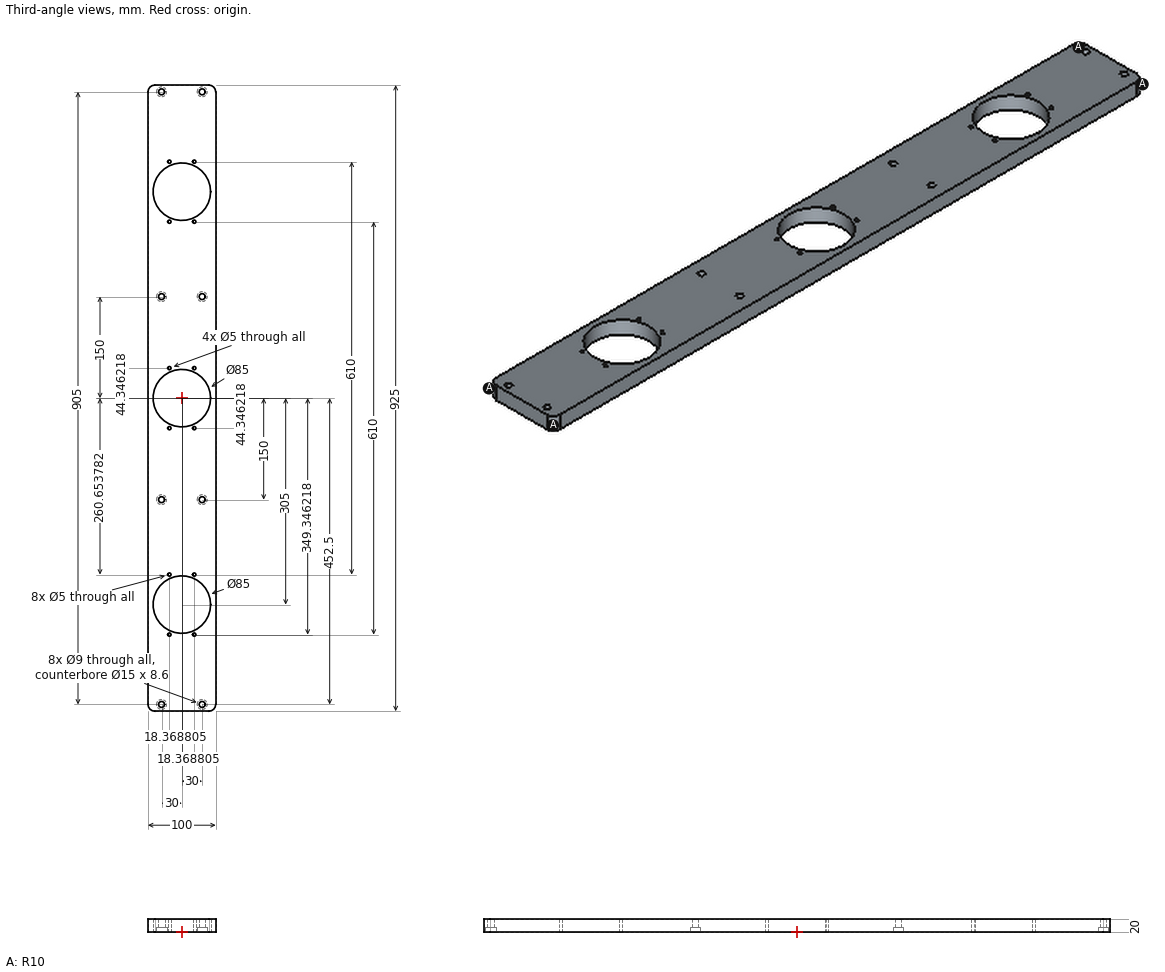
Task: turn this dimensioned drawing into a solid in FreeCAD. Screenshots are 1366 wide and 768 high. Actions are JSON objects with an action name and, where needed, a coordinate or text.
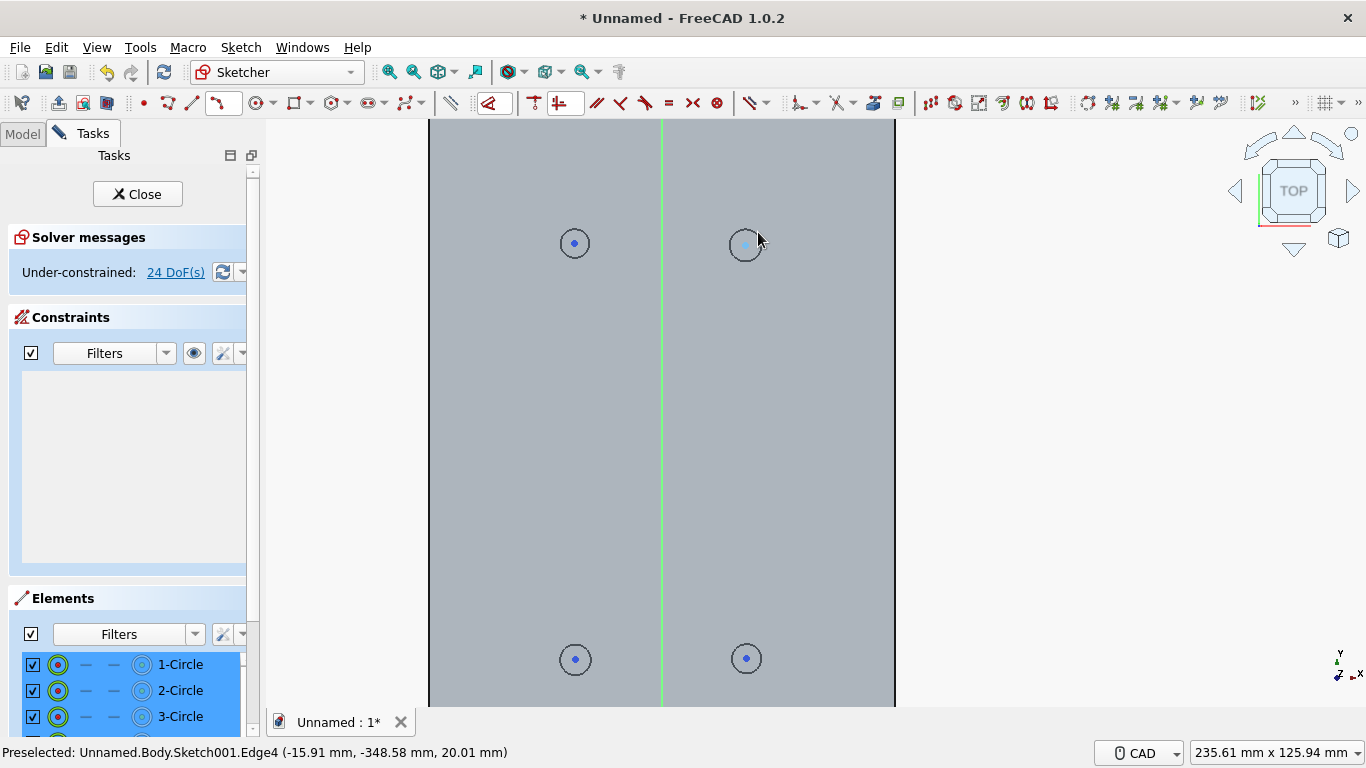
{"action": "left_click", "coordinate": [757, 234]}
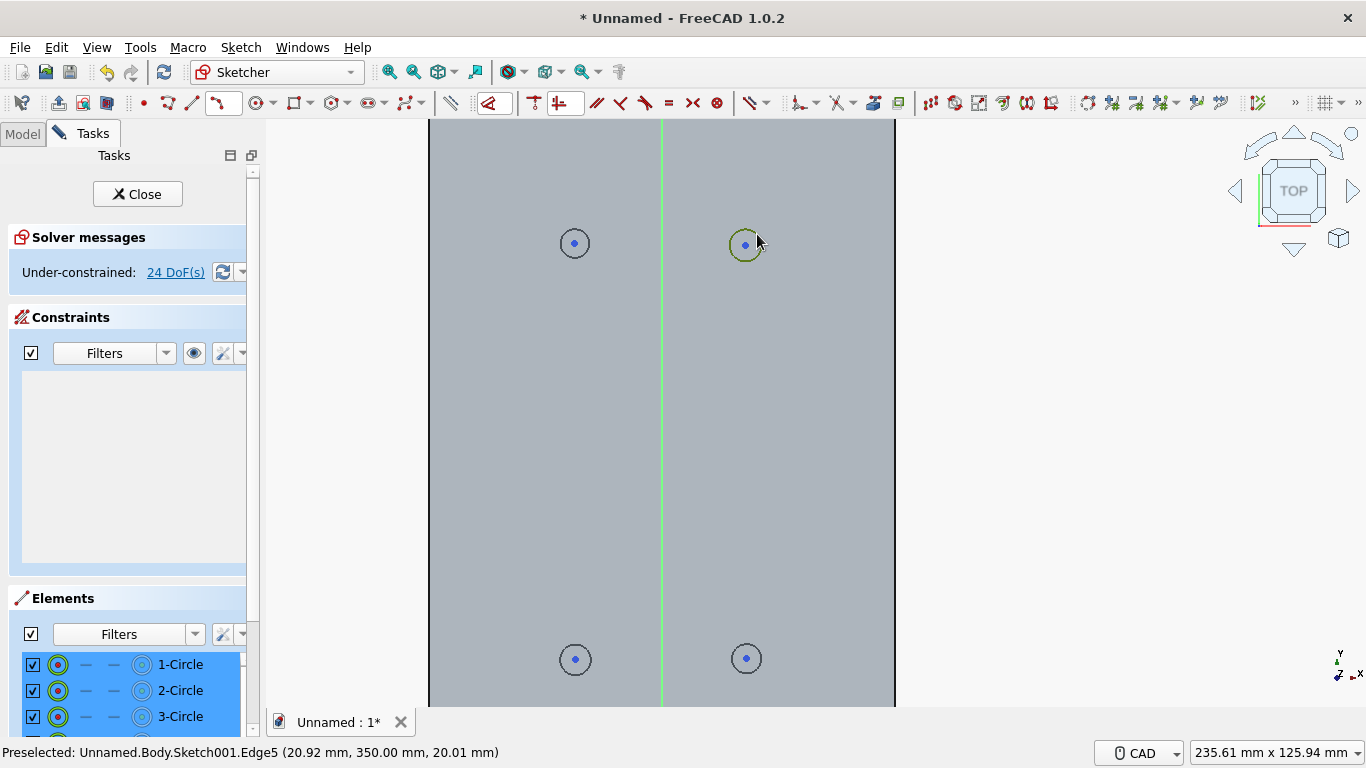
{"action": "left_click", "coordinate": [585, 233]}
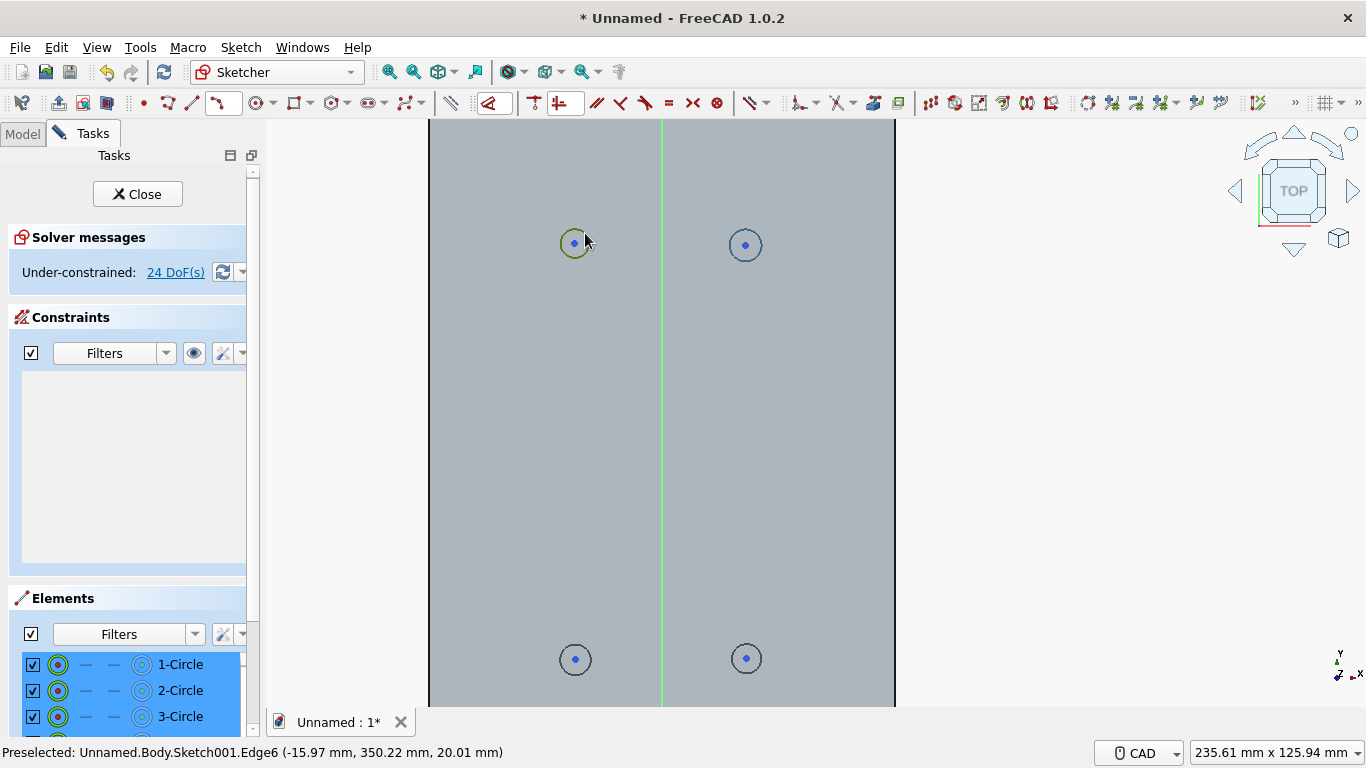
{"action": "left_click", "coordinate": [757, 648]}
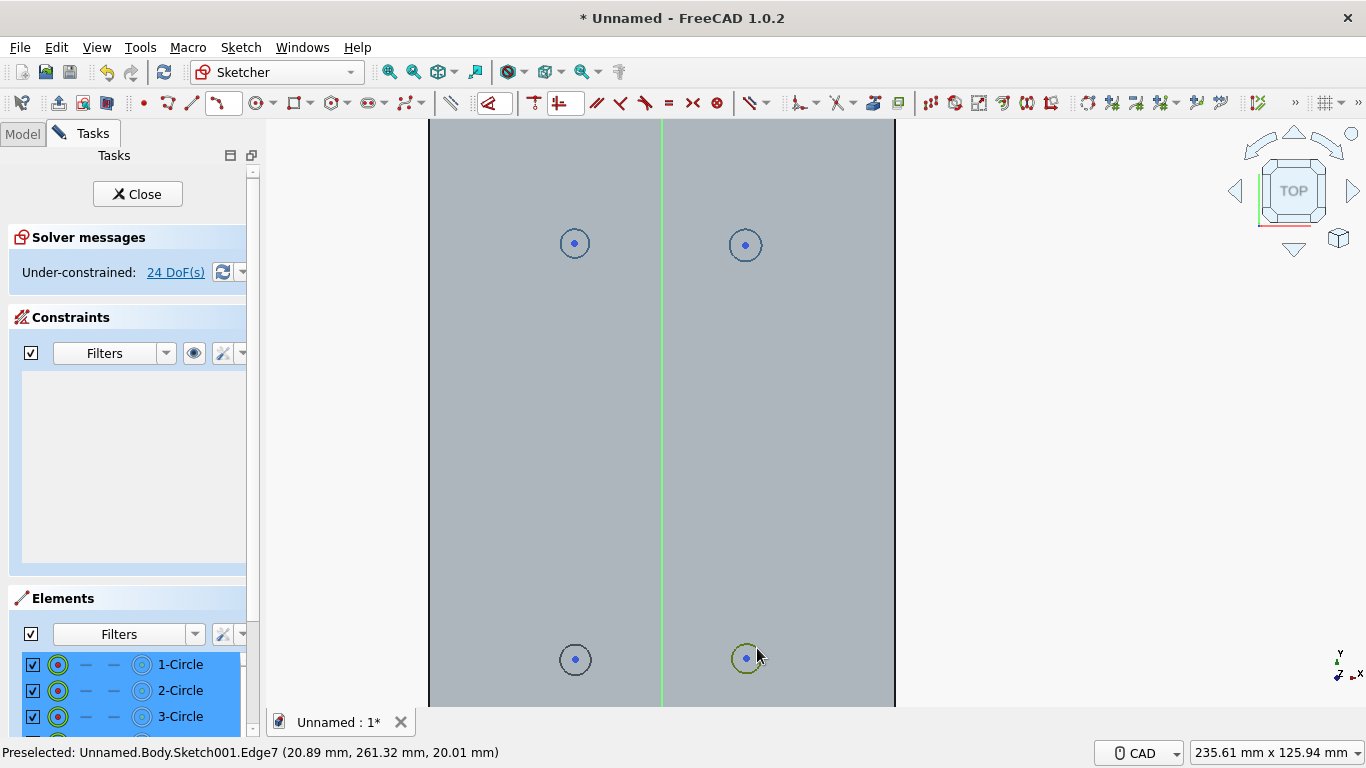
{"action": "left_click", "coordinate": [586, 649]}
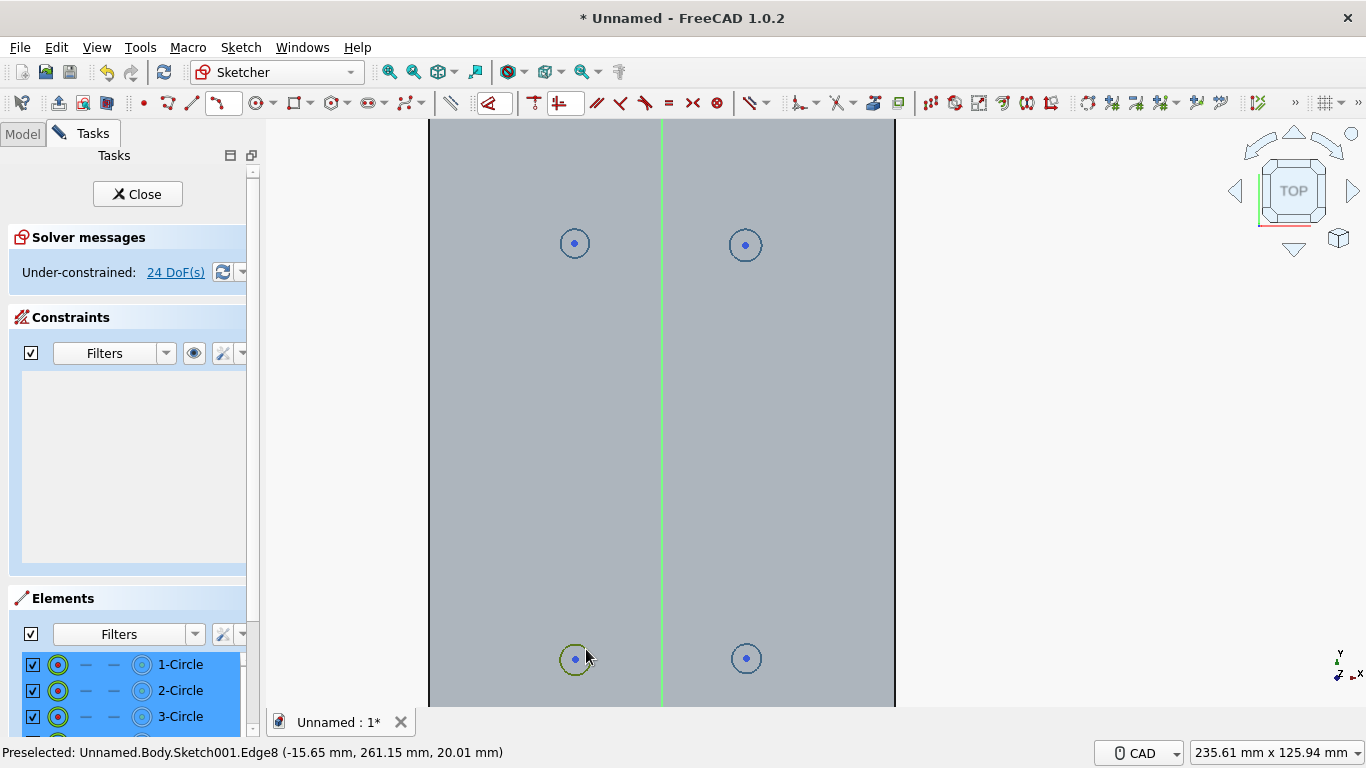
{"action": "key", "text": "e"}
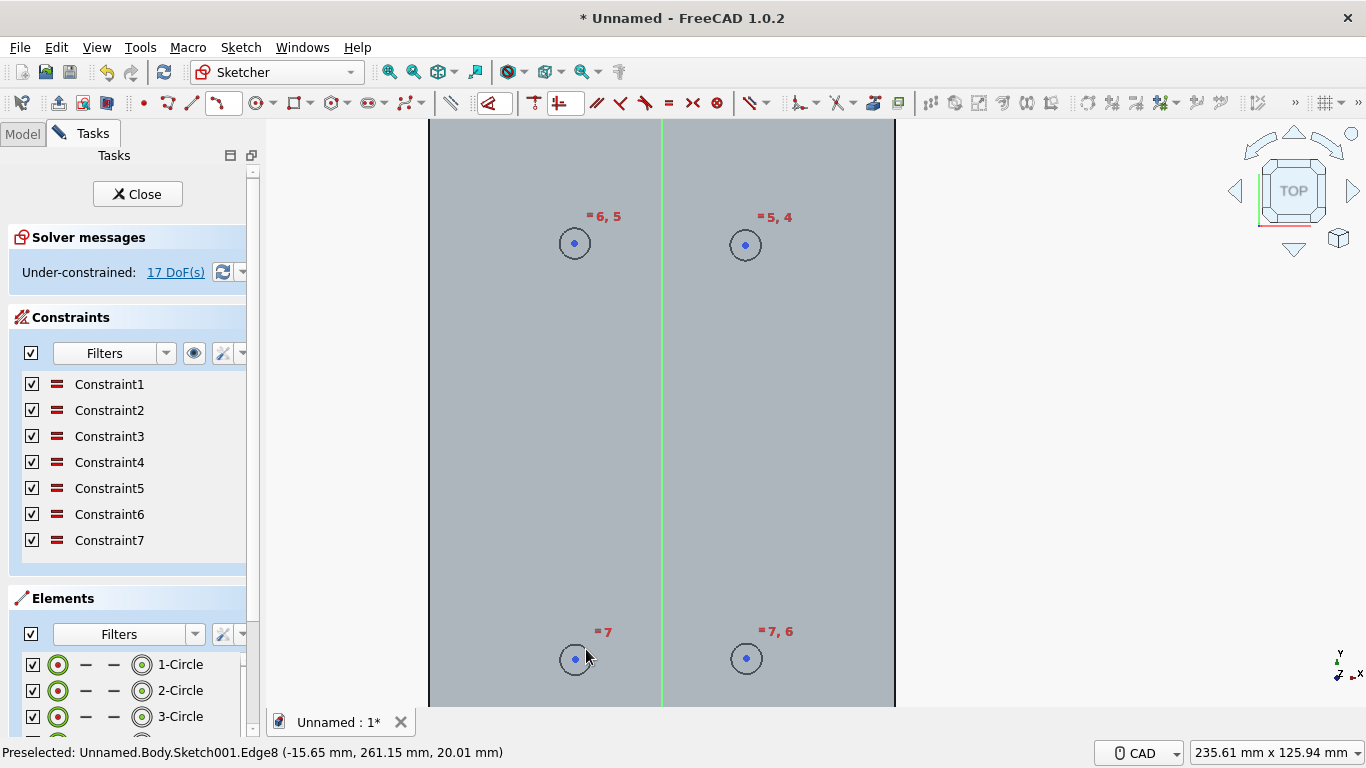
{"action": "key", "text": "d"}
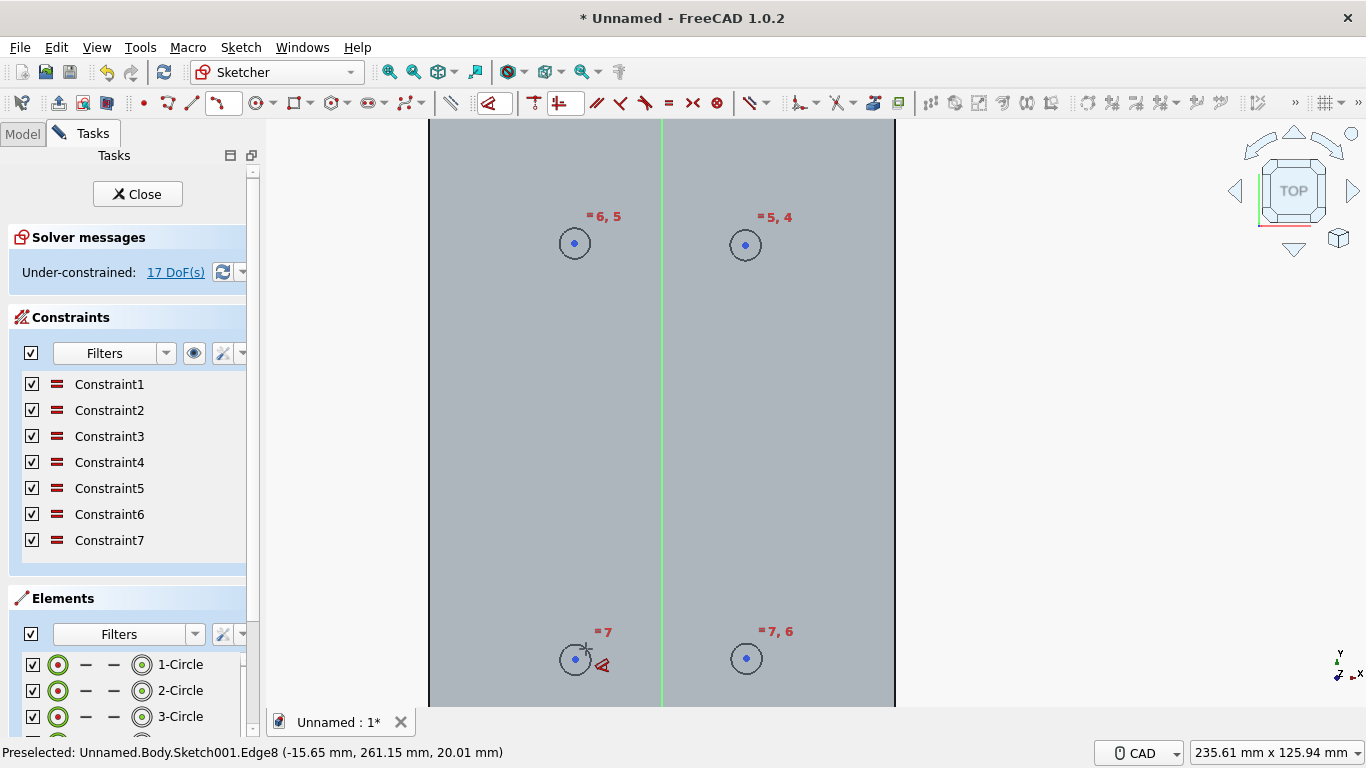
{"action": "scroll", "coordinate": [758, 231], "scroll_direction": "down", "scroll_amount": 11}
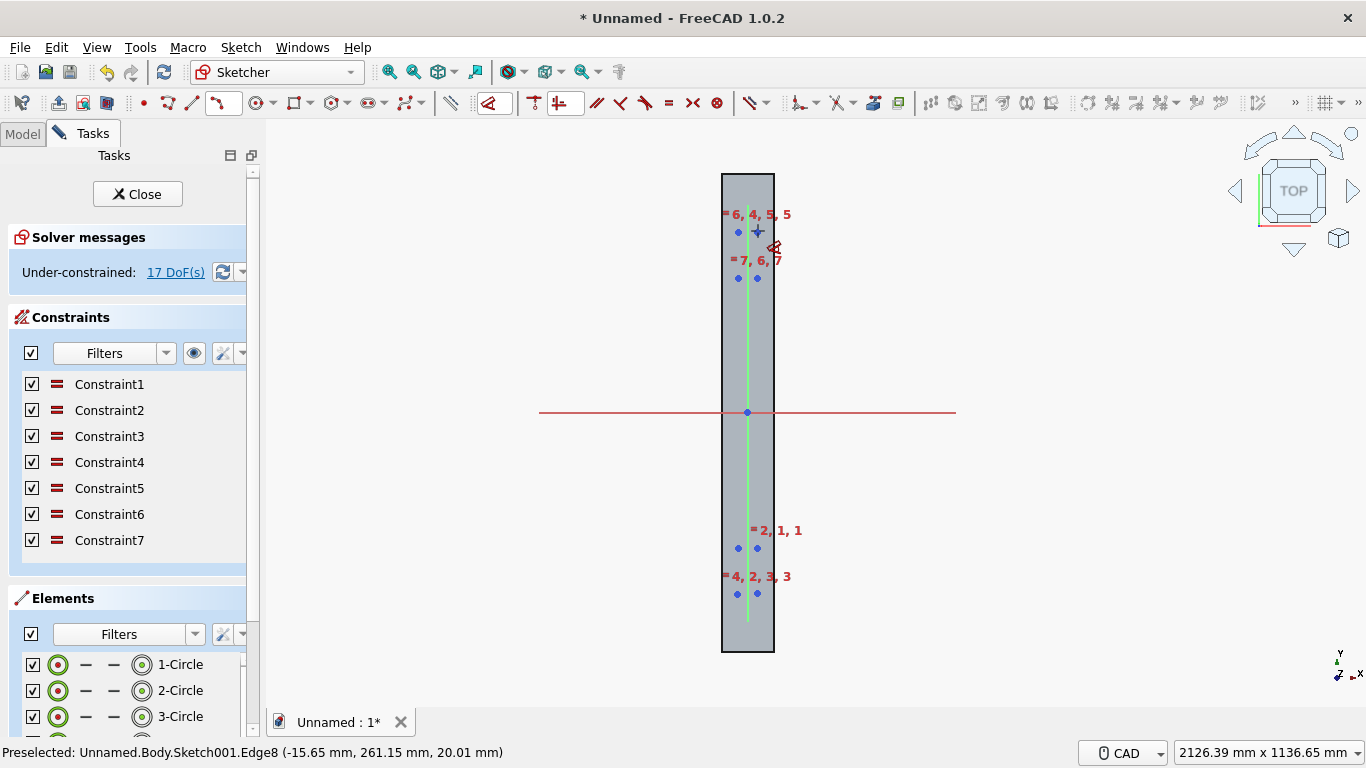
{"action": "scroll", "coordinate": [739, 547], "scroll_direction": "up", "scroll_amount": 14}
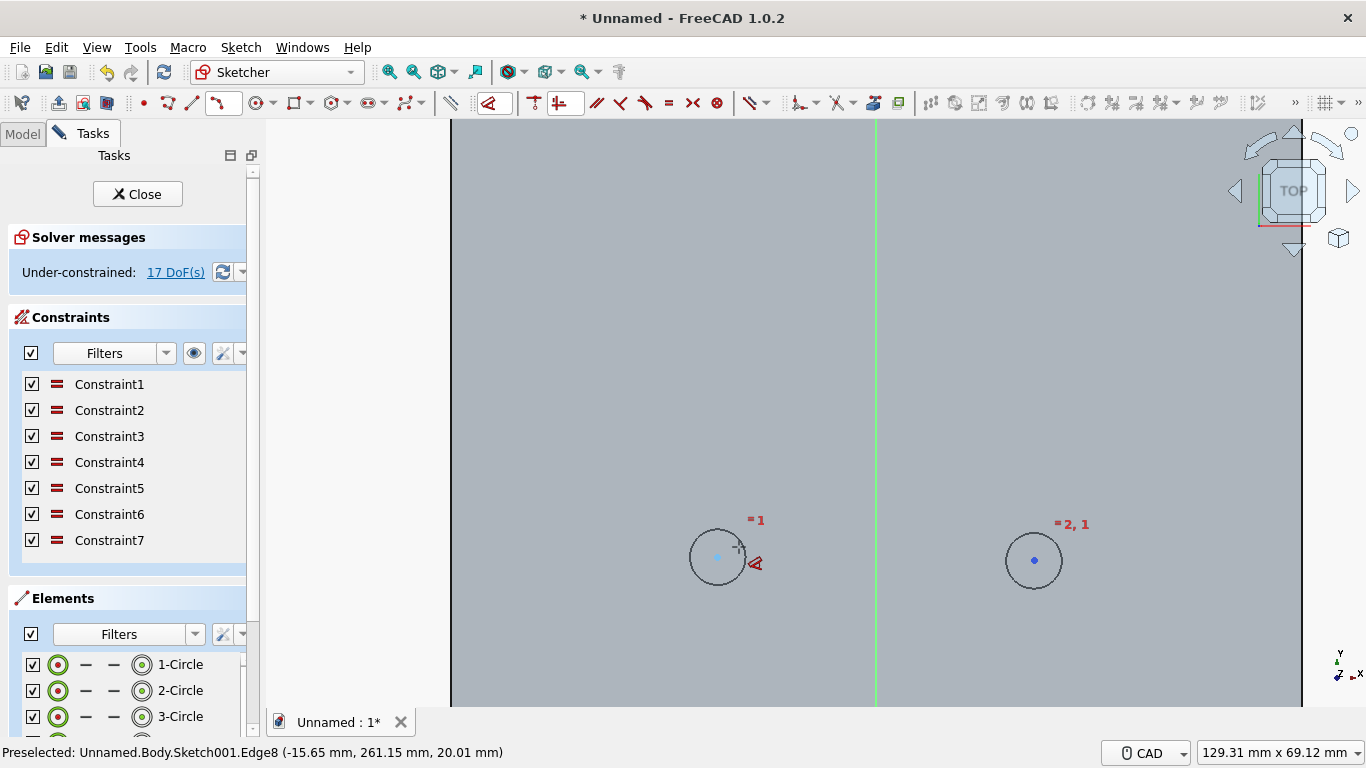
{"action": "left_click", "coordinate": [737, 537]}
{"action": "left_click", "coordinate": [759, 514]}